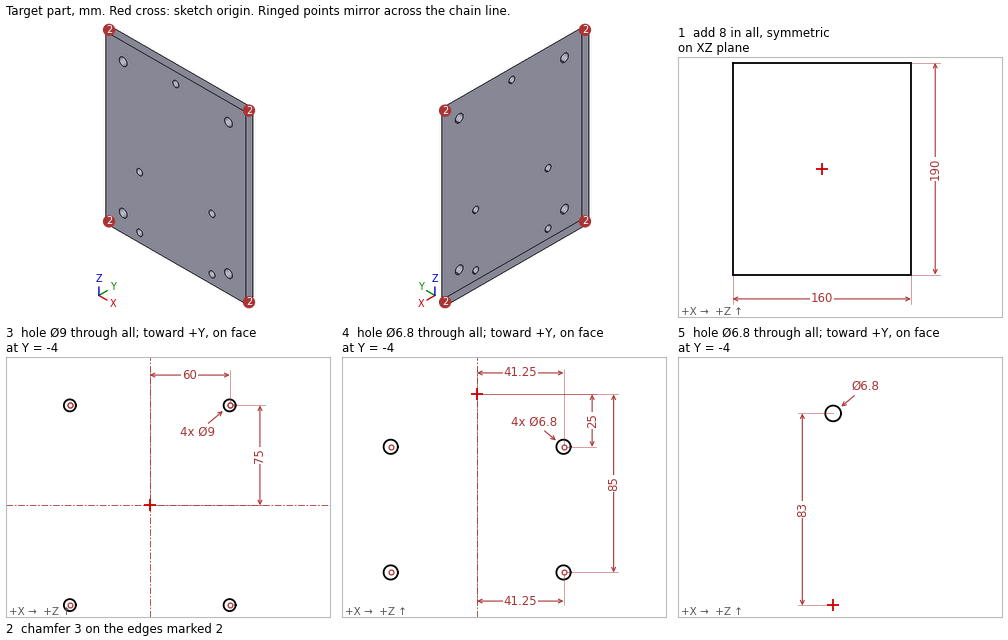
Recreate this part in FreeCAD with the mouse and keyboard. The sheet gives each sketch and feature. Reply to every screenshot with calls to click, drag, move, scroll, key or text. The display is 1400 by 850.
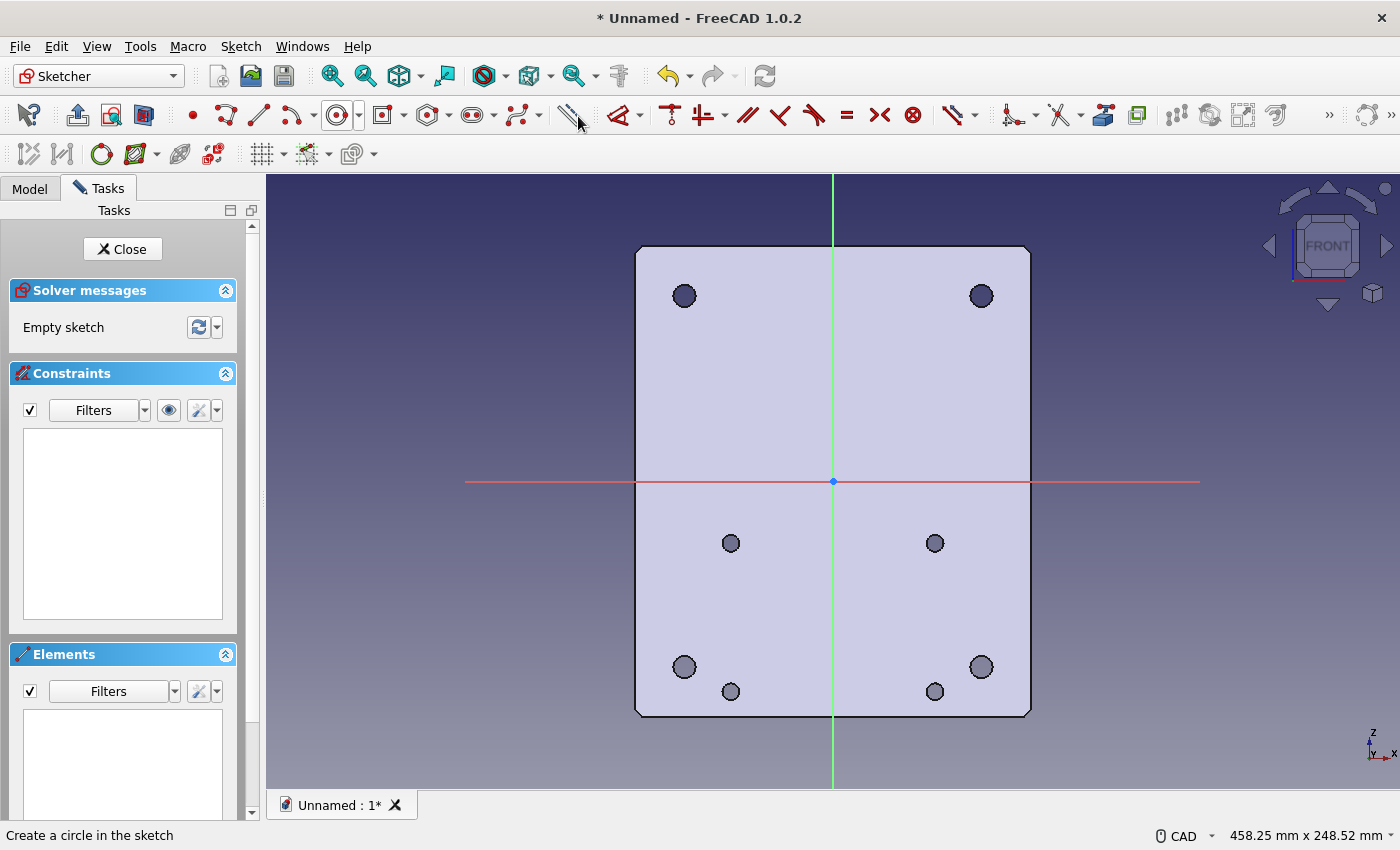
scroll(837, 265, up, 15)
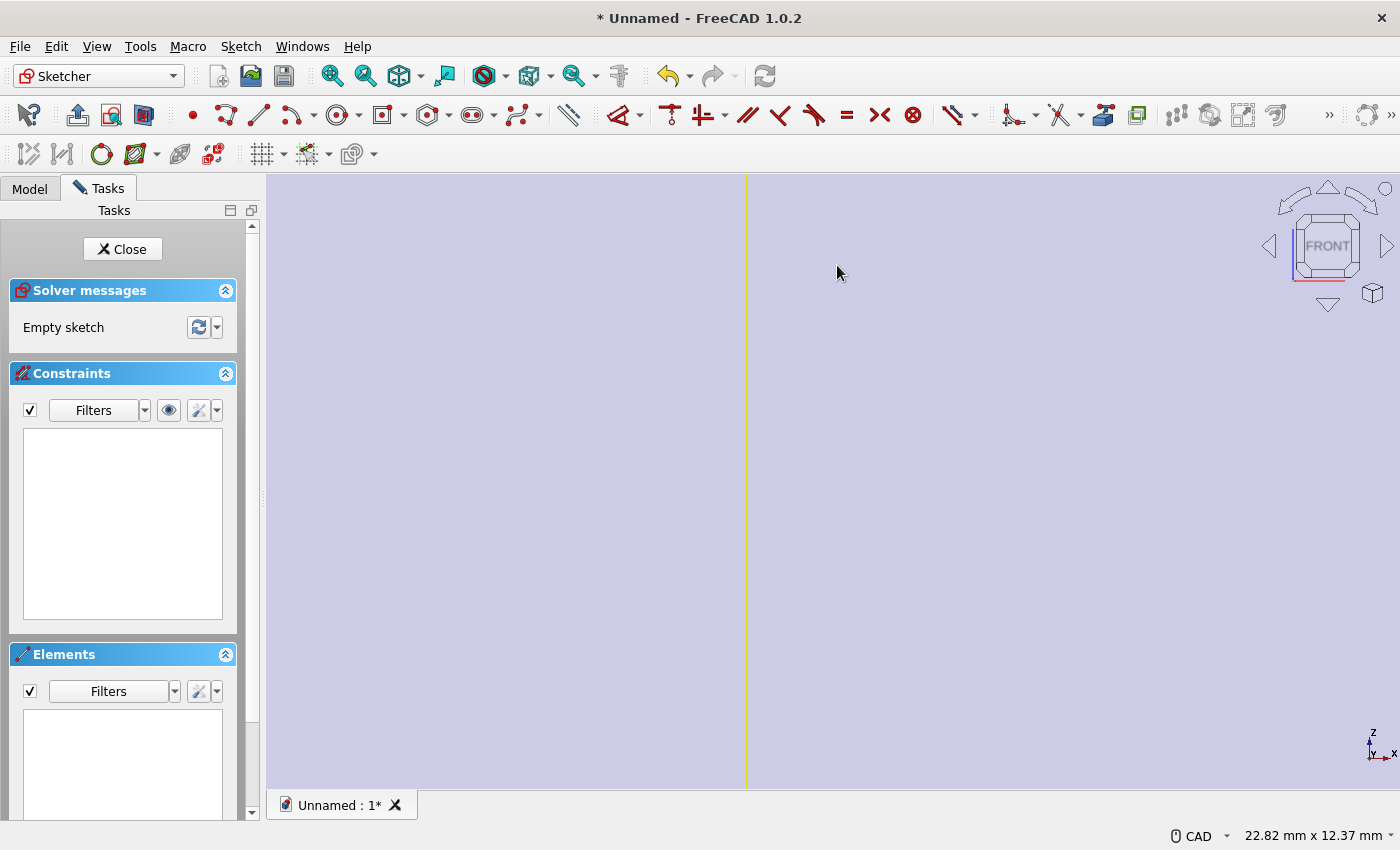
click(336, 116)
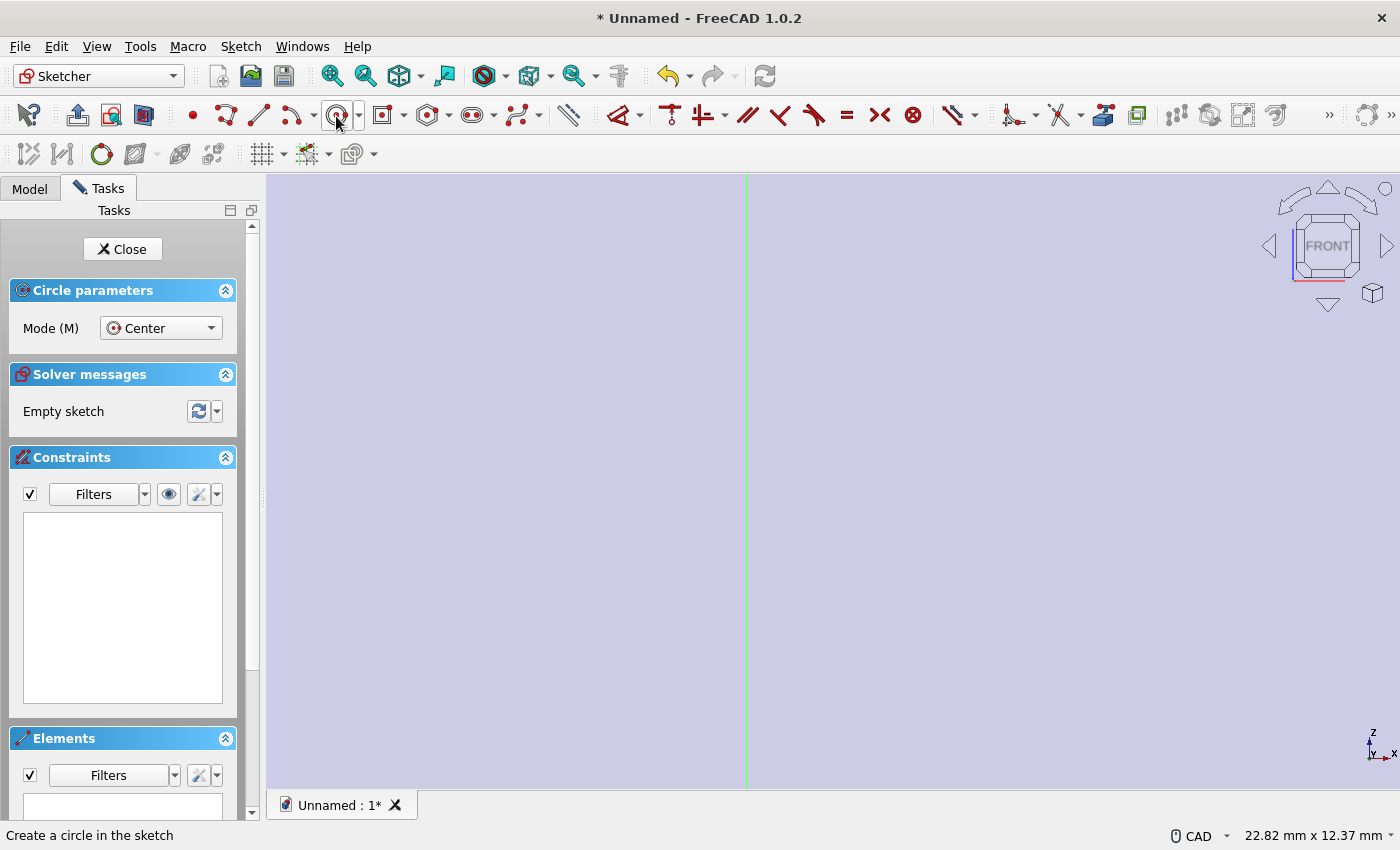
click(747, 485)
click(867, 366)
key(Escape)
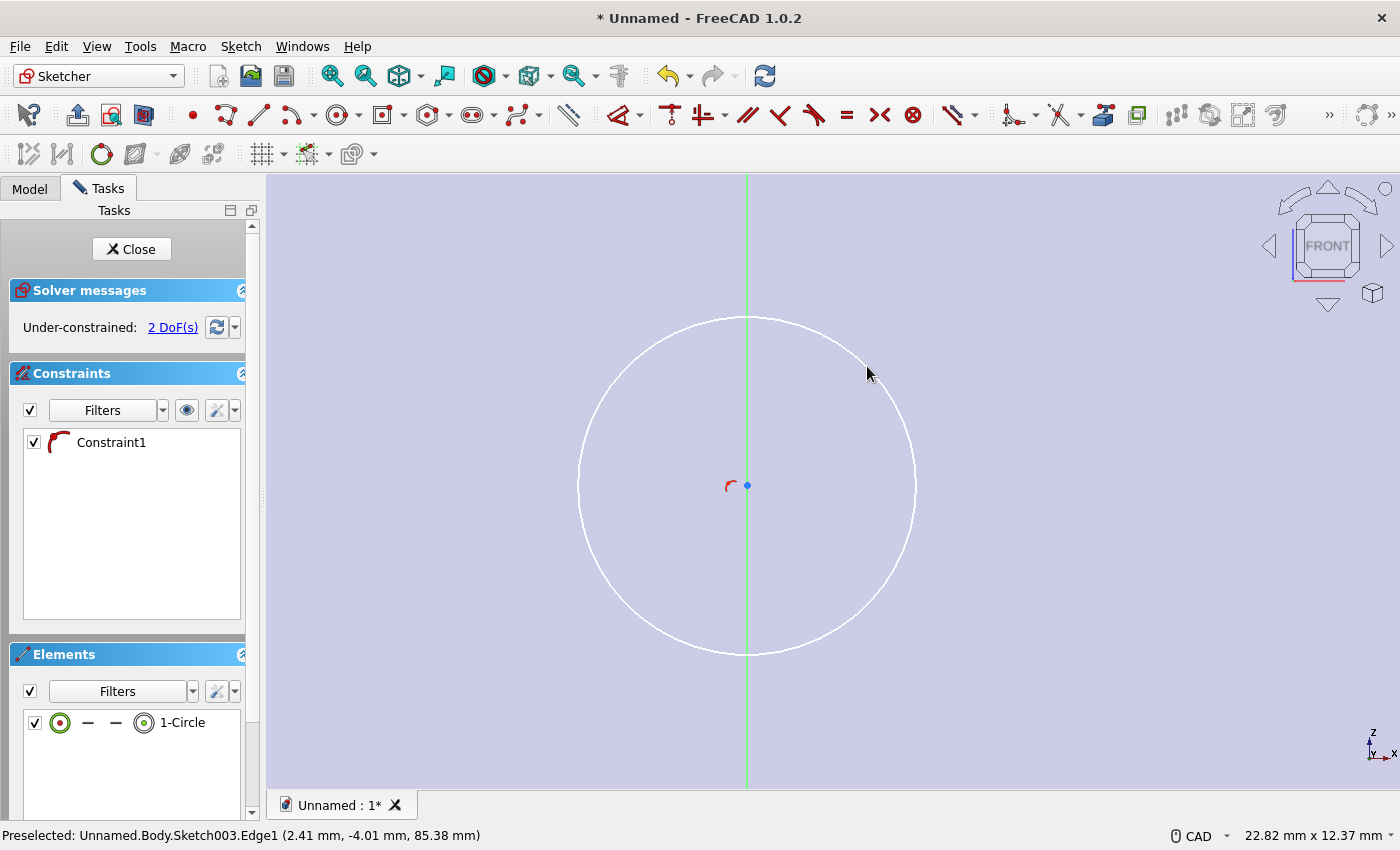
key(d)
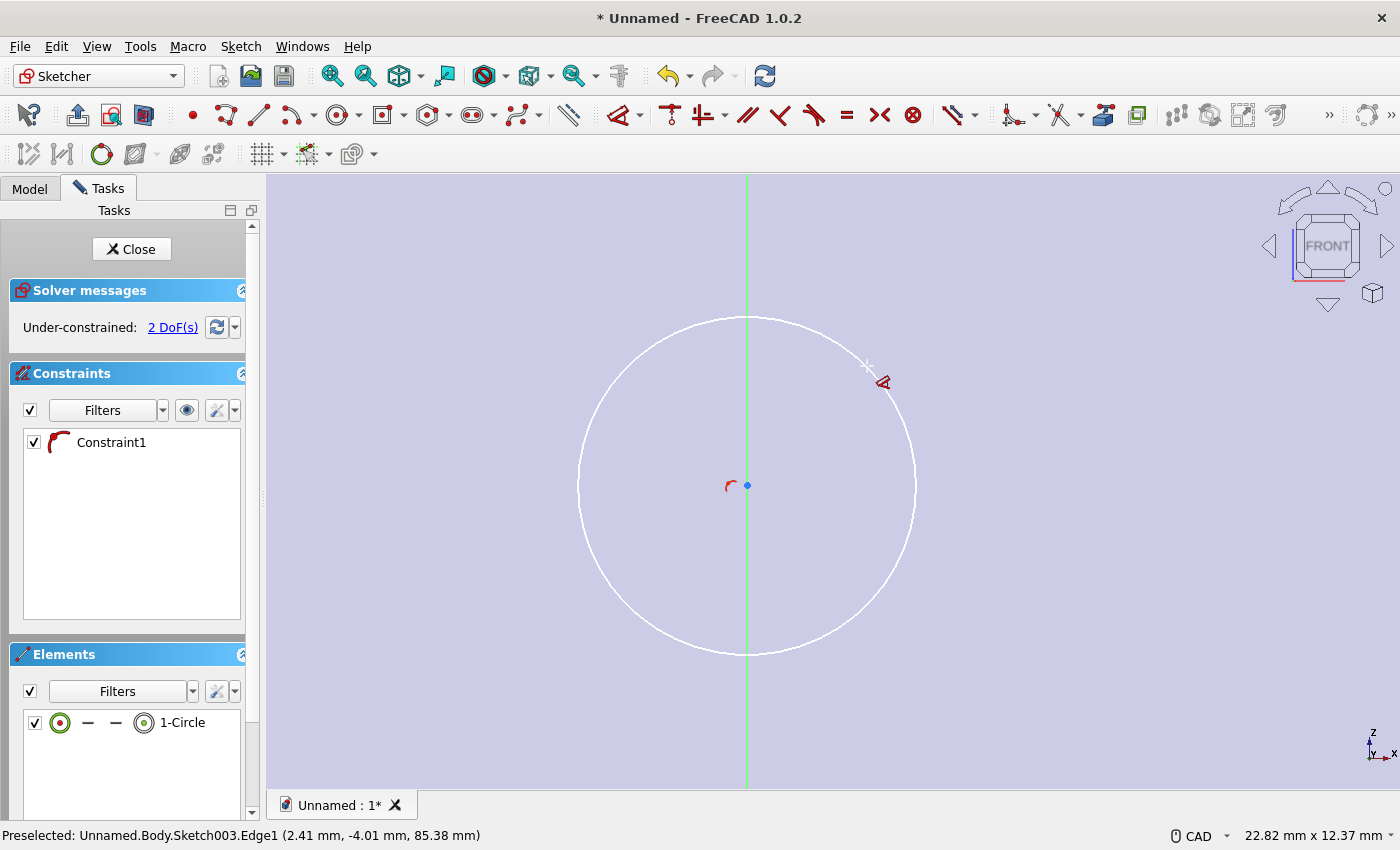
click(866, 366)
click(889, 343)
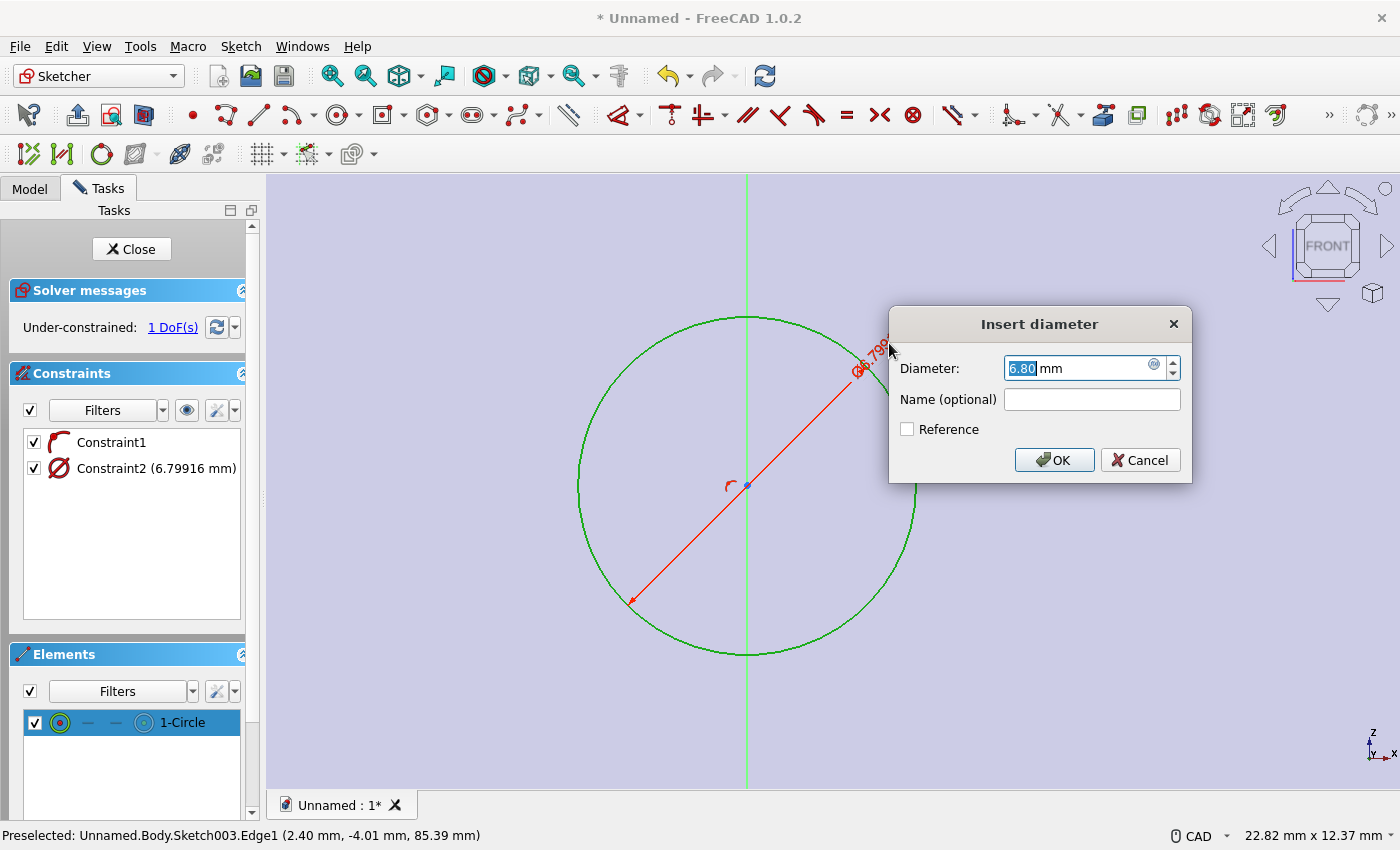
text(6.8)
key(Return)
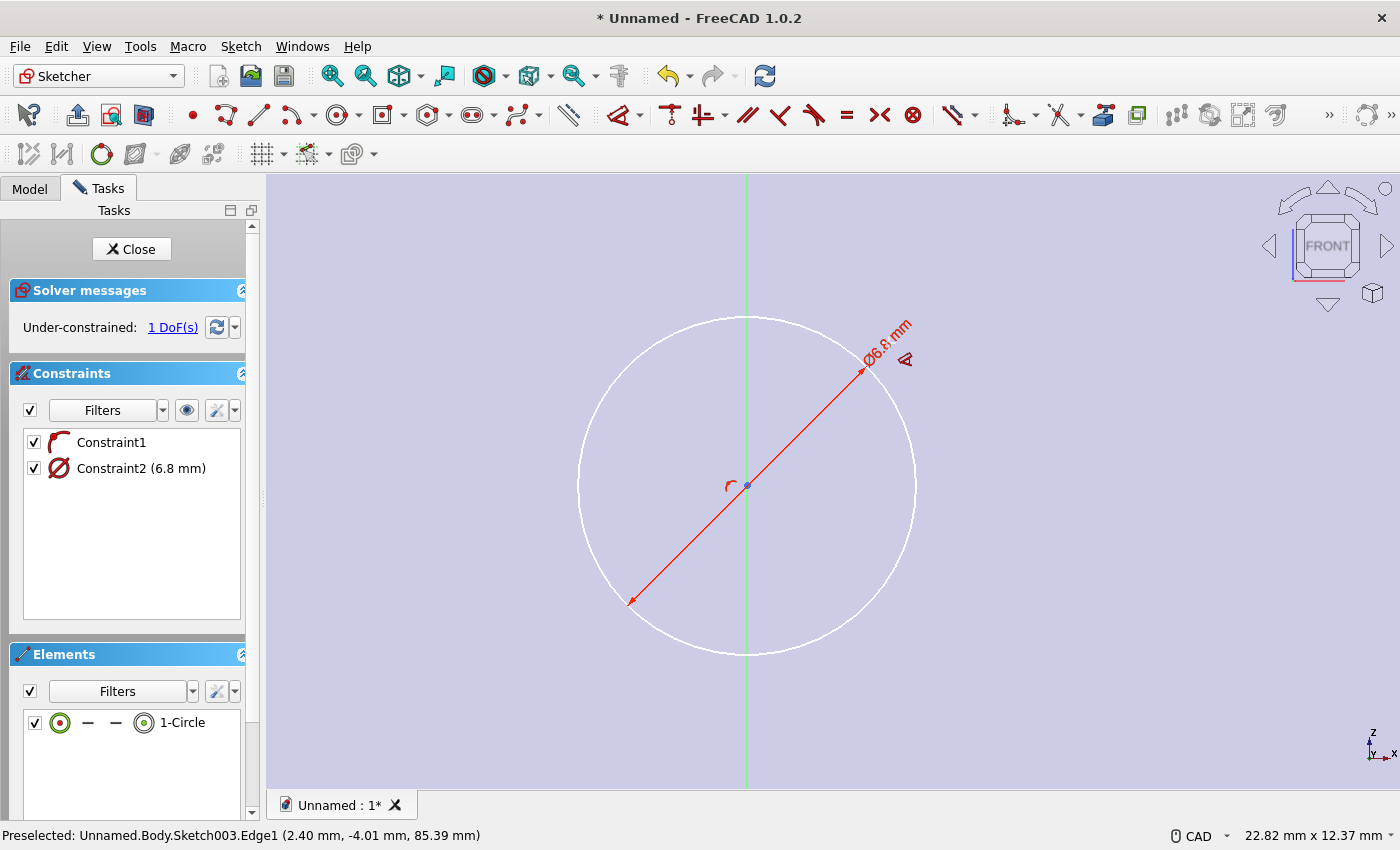
click(747, 486)
click(781, 624)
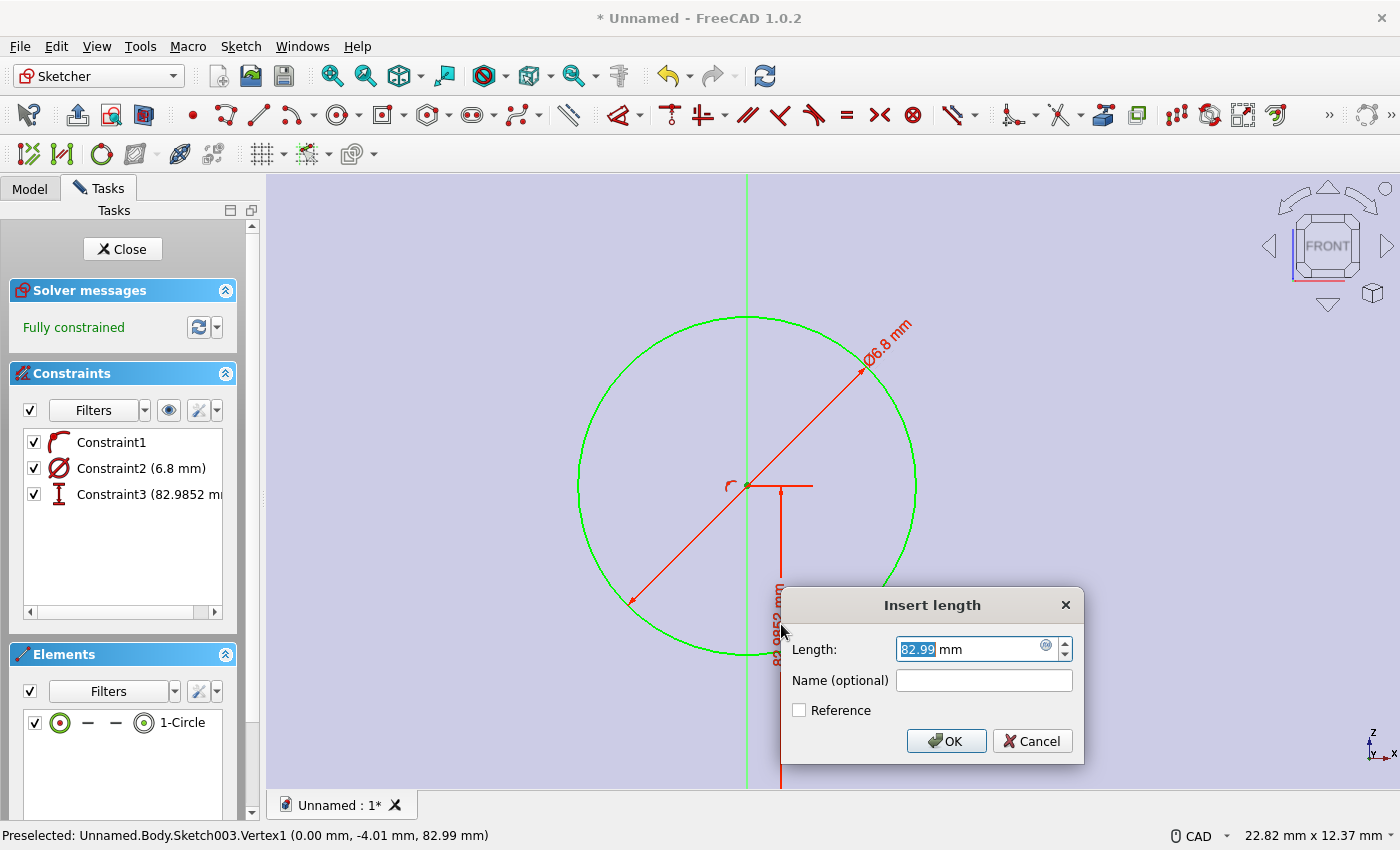
text(83)
key(Return)
key(Escape)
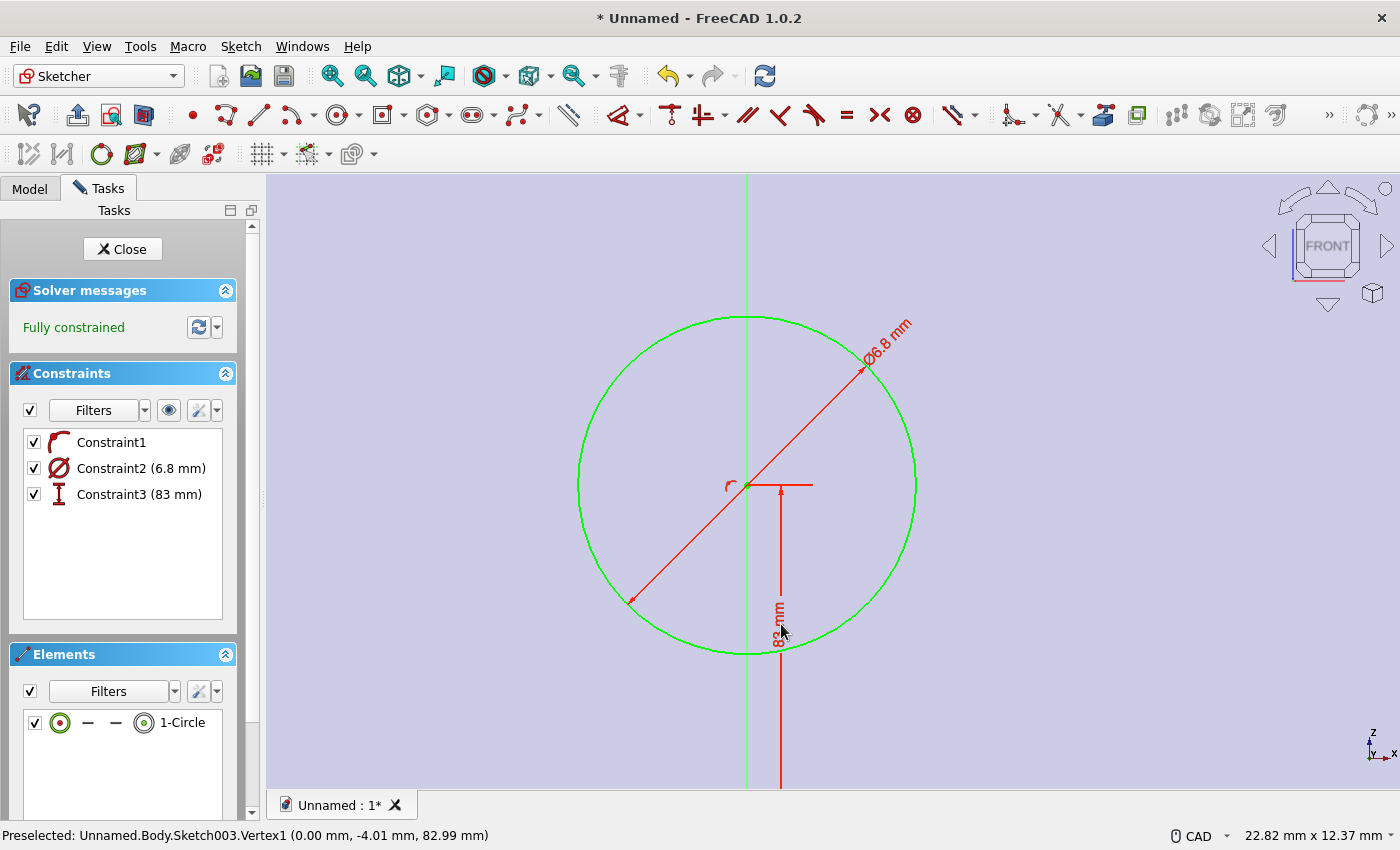
click(123, 249)